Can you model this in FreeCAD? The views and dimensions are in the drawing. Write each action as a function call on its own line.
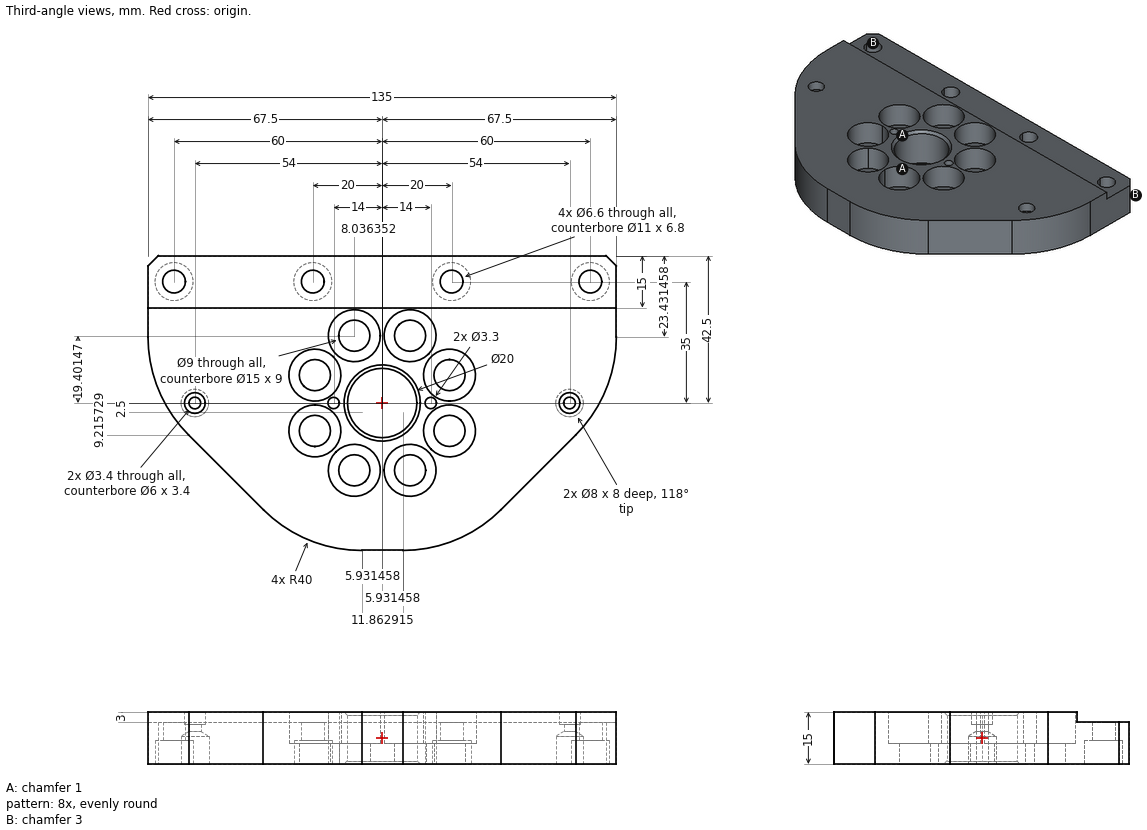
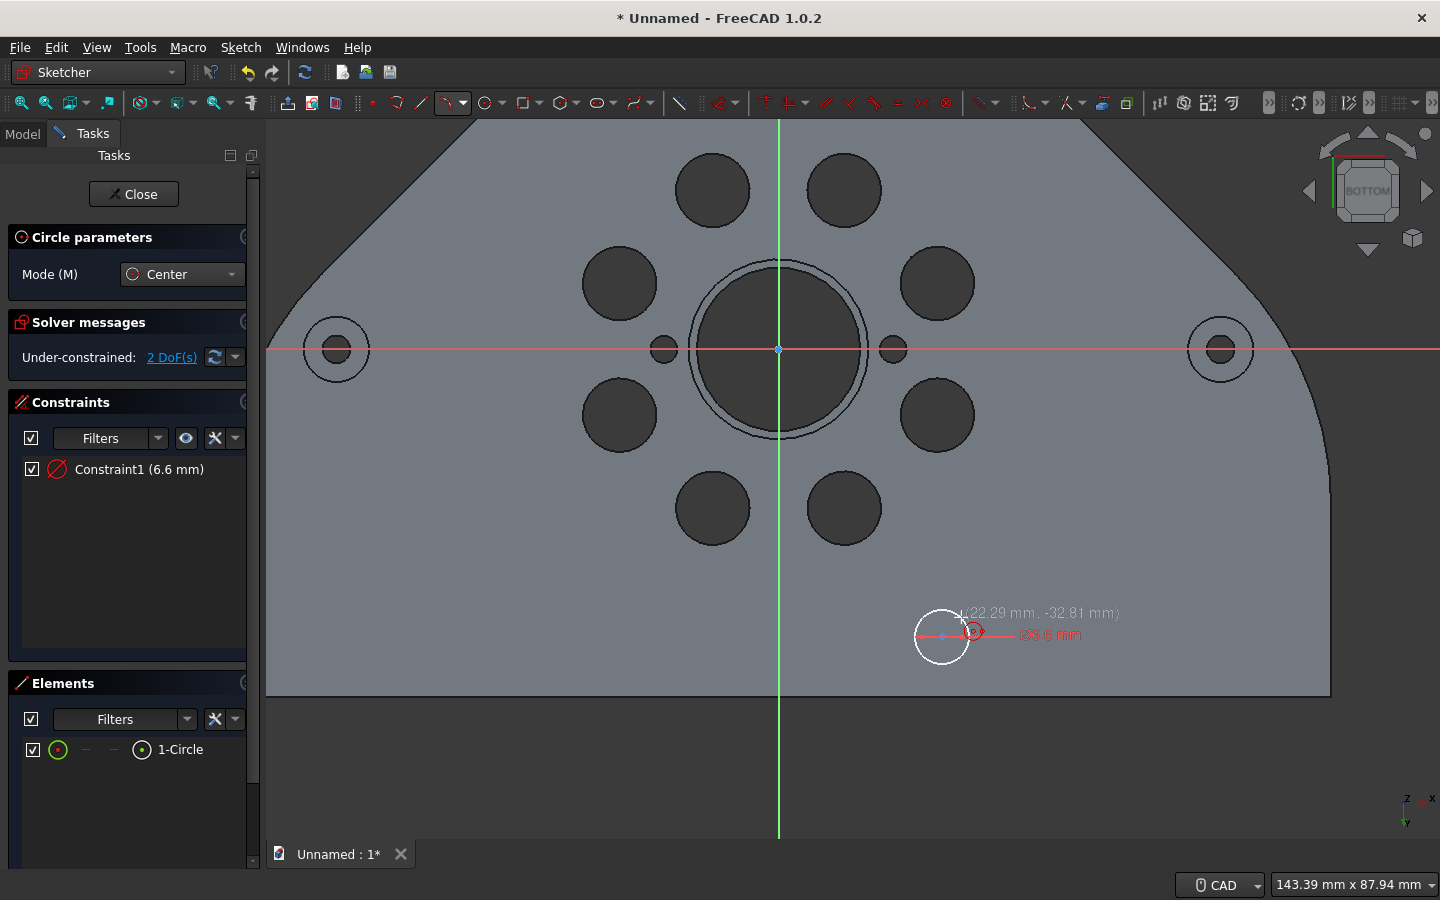
click(1270, 636)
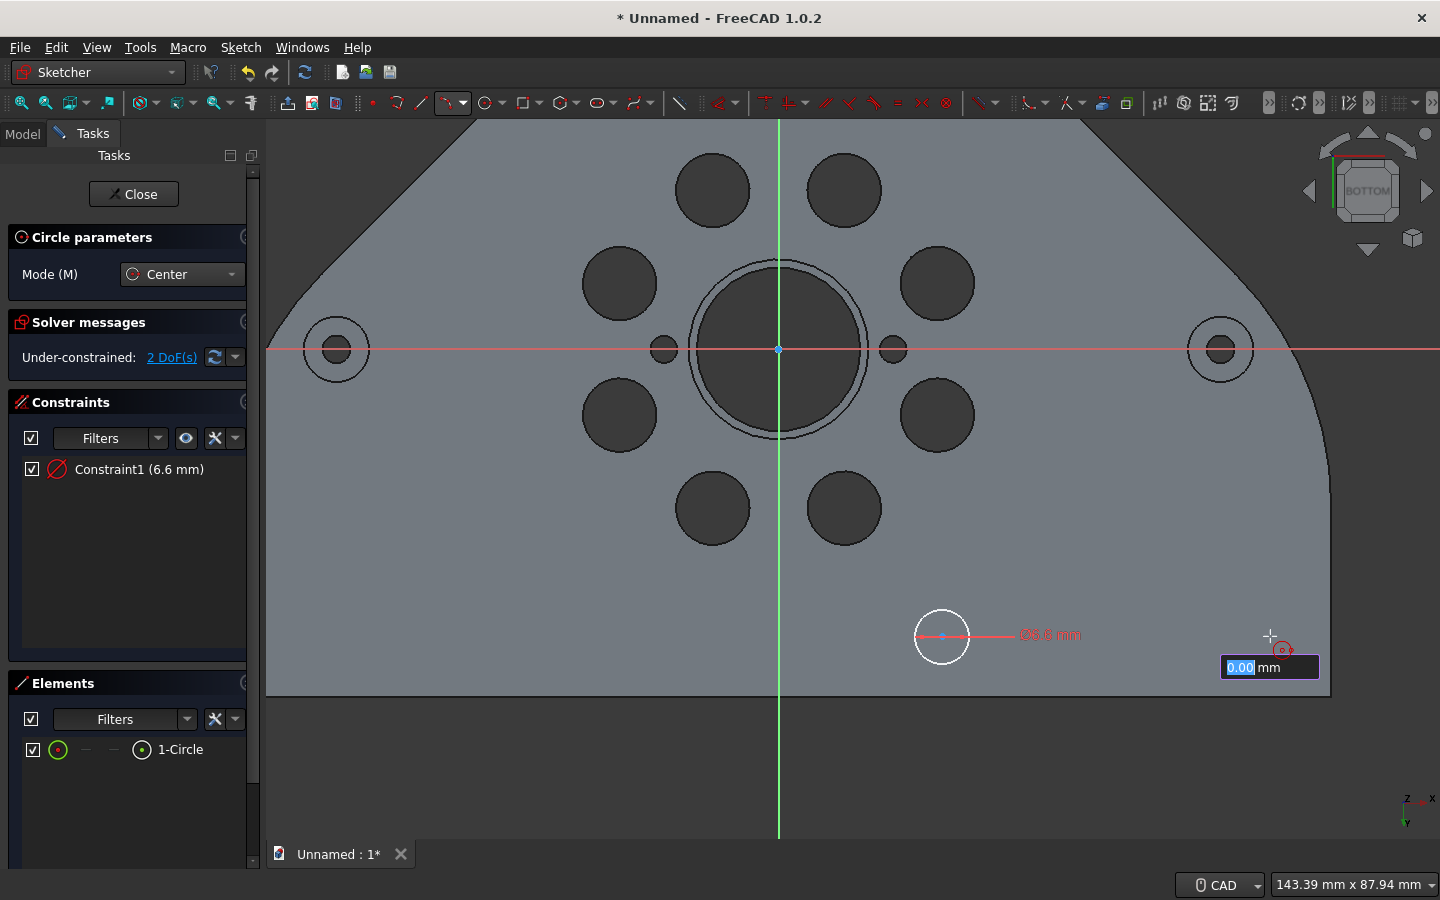
scroll(797, 424, down, 2)
move(1127, 553)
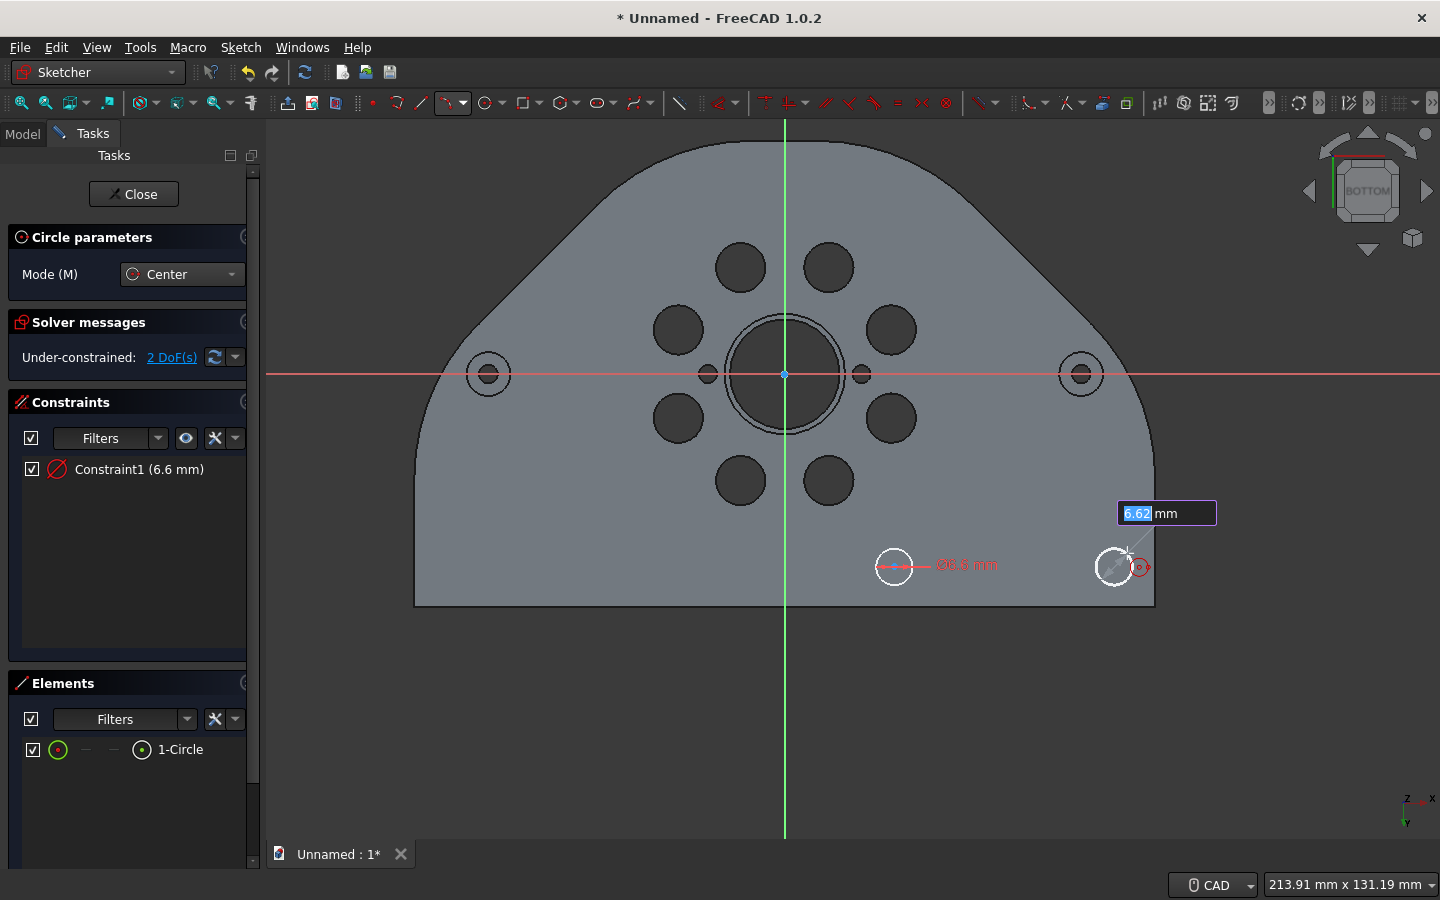
text(6.6)
key(Return)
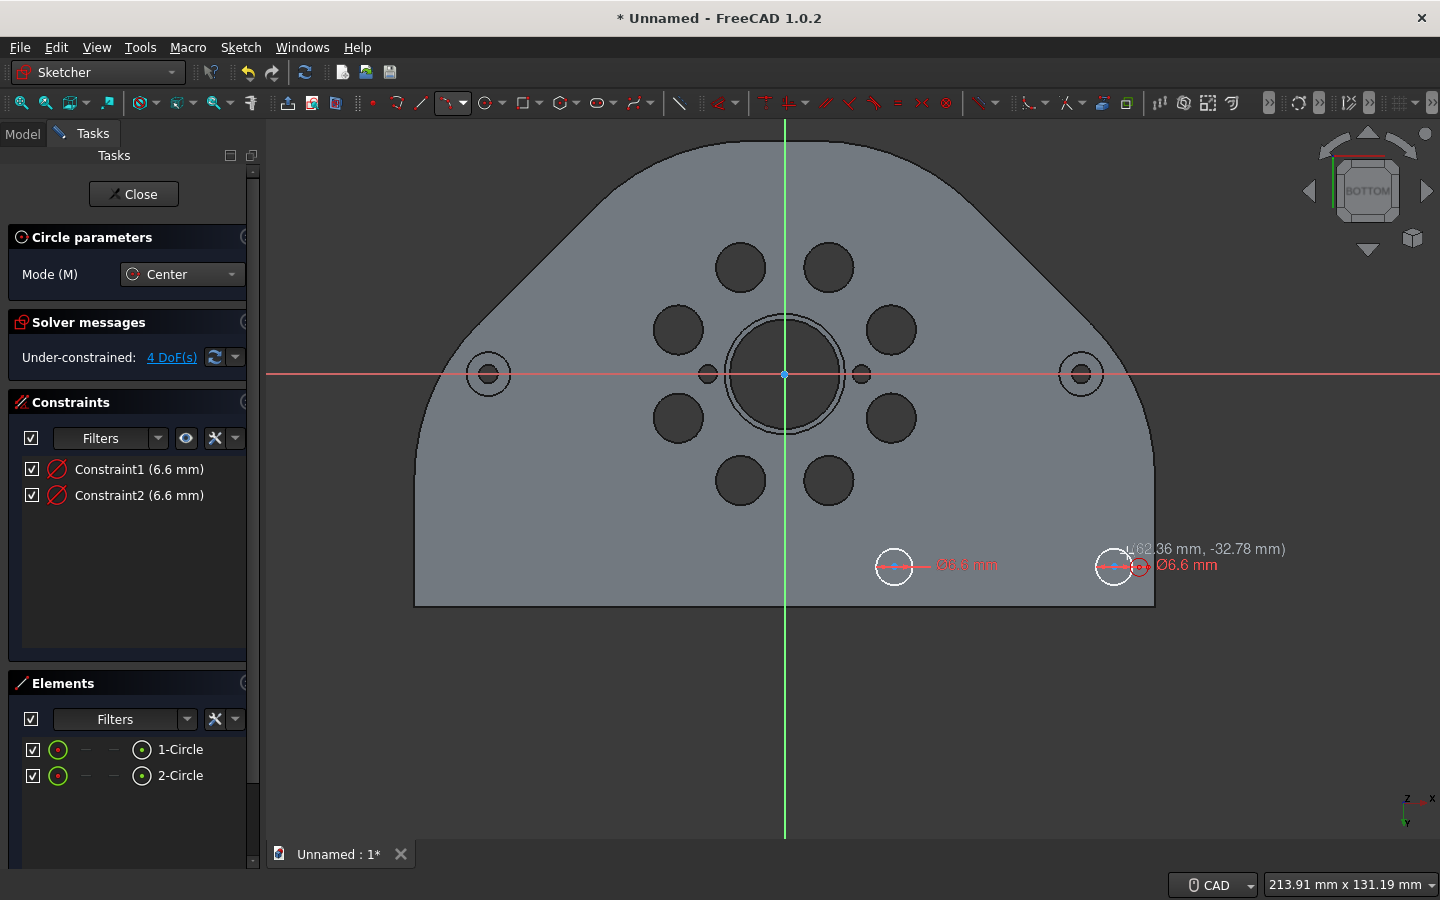
scroll(455, 566, up, 2)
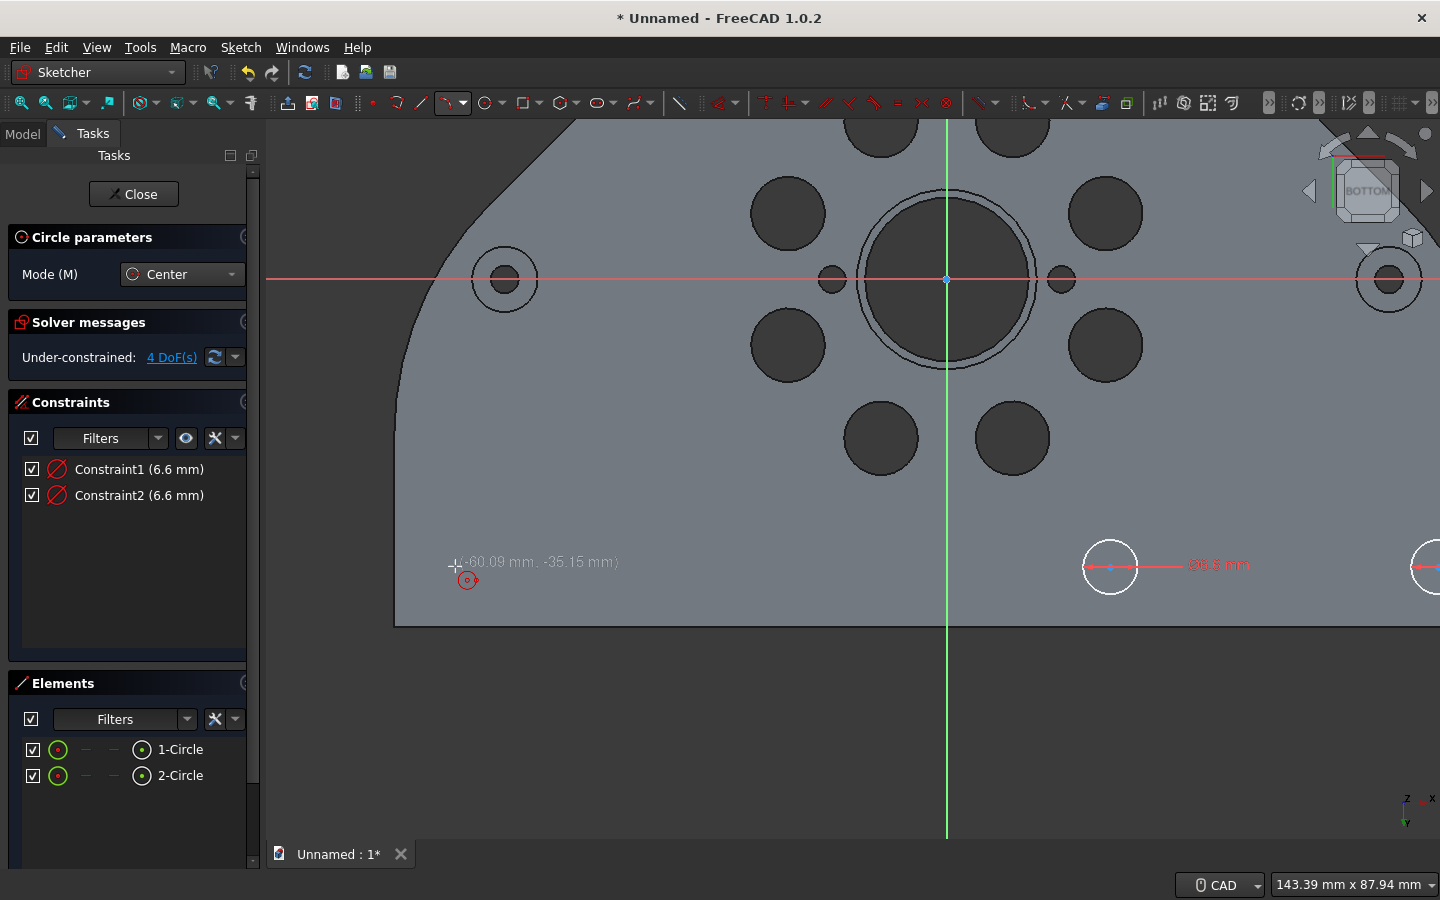
click(456, 566)
move(475, 547)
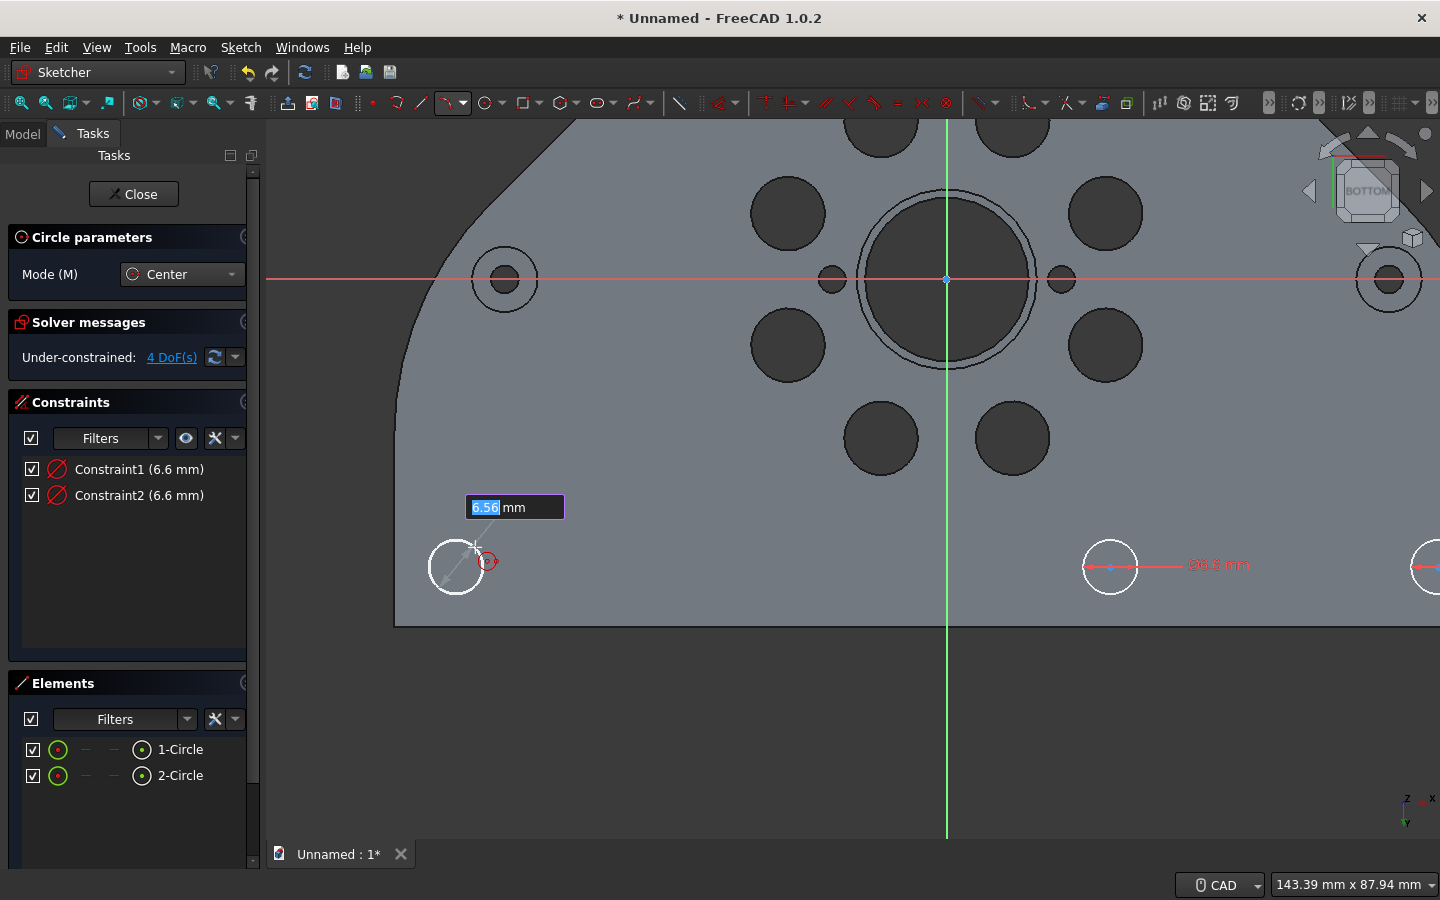
text(6.6)
key(Return)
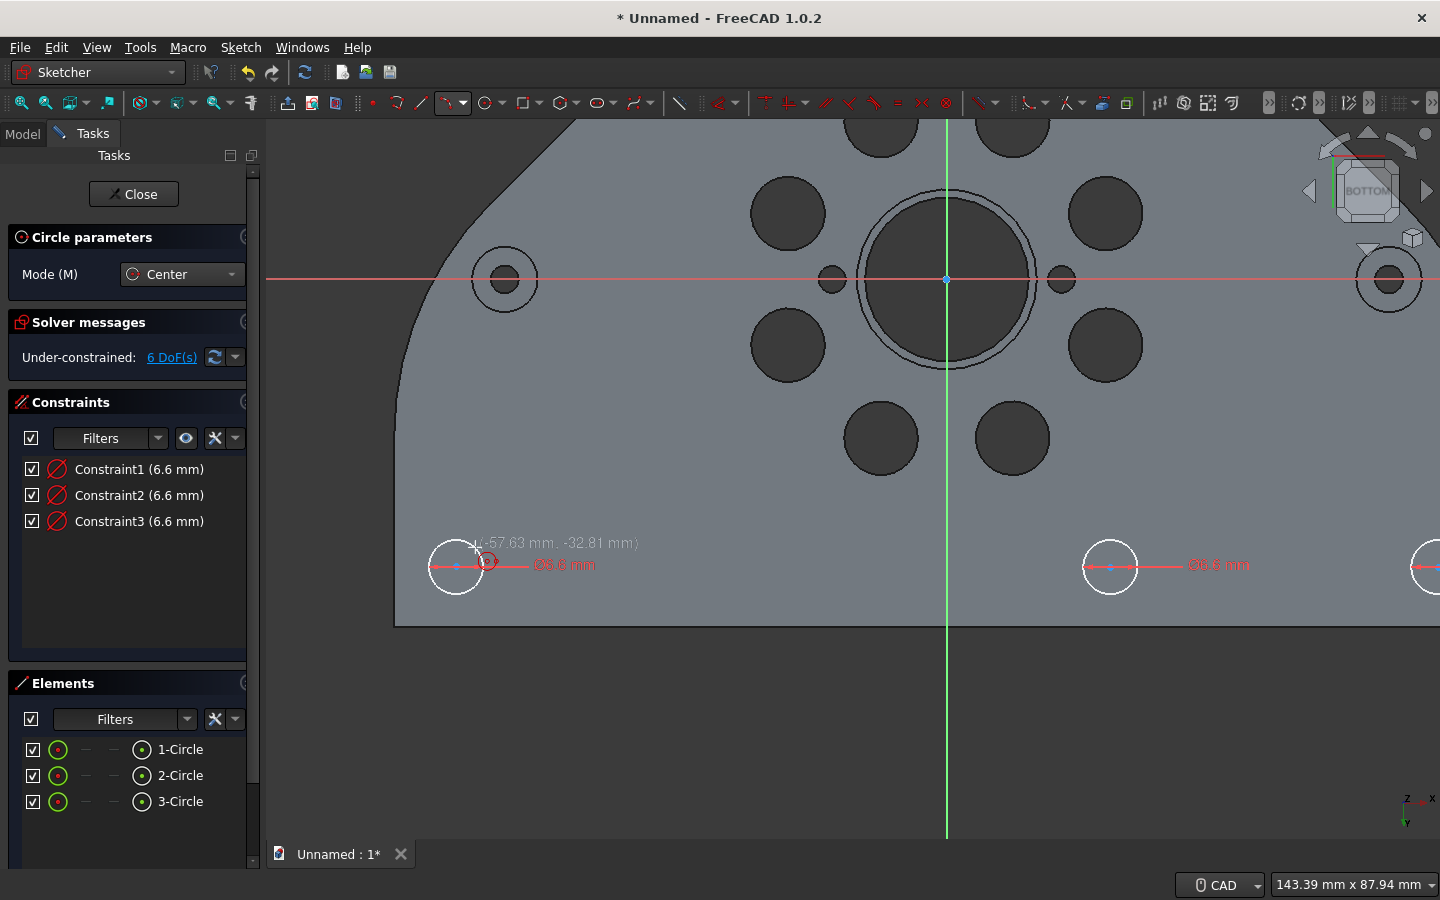
click(783, 566)
move(802, 547)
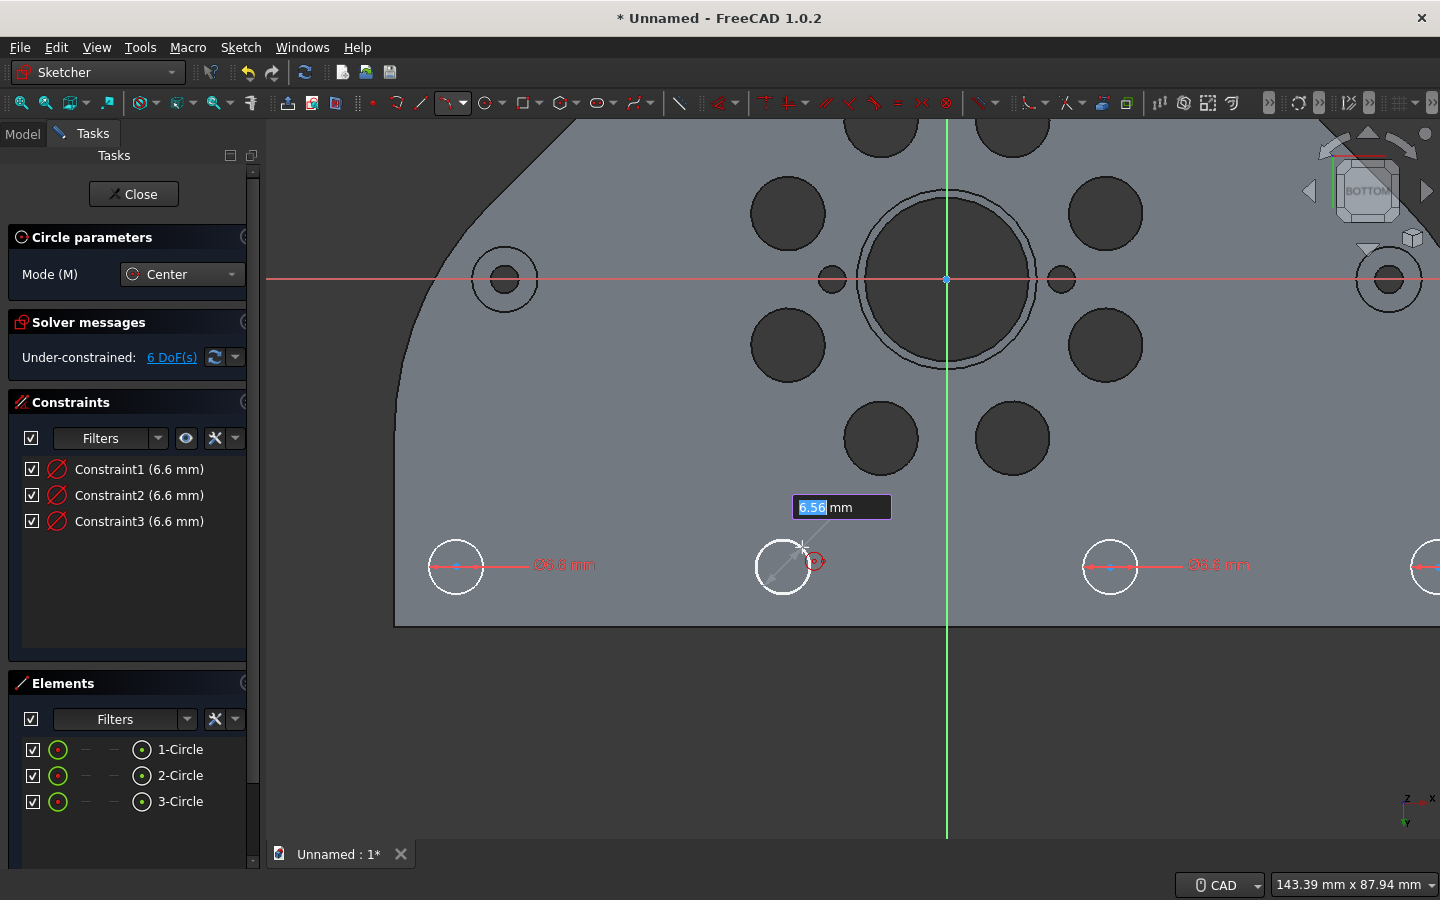
text(6.6)
key(Return)
key(Escape)